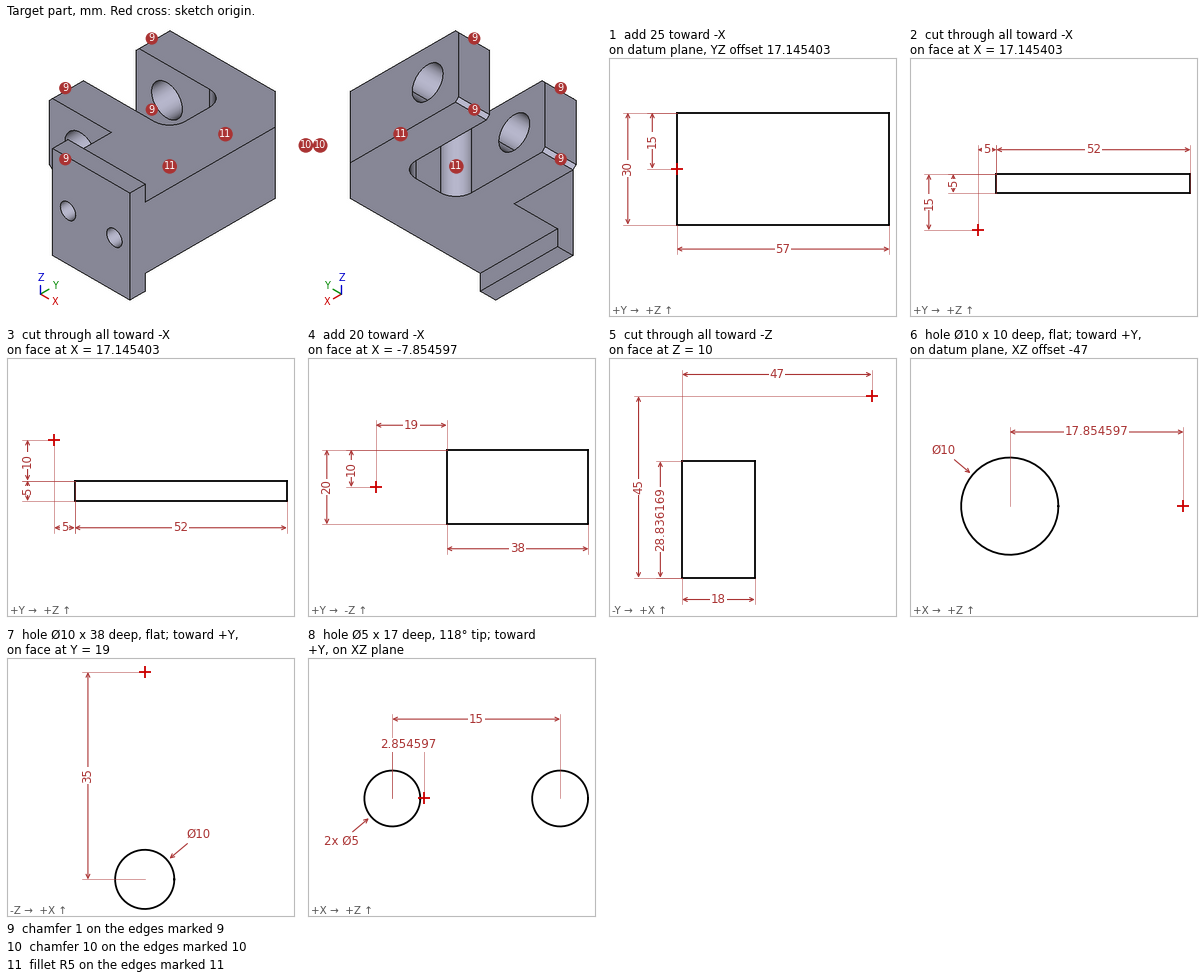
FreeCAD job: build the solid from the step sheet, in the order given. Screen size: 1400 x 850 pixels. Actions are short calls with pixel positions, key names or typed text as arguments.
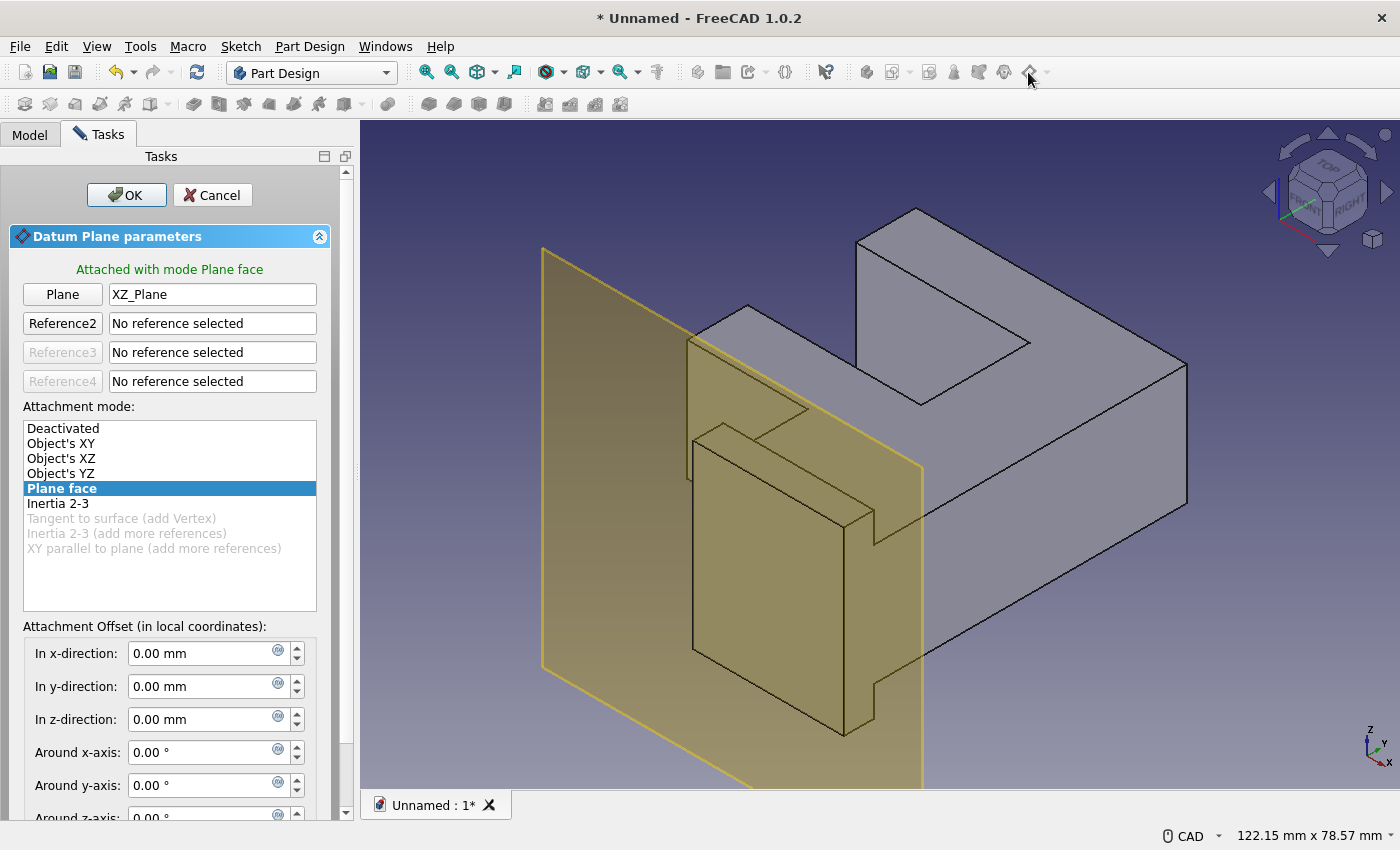
triple_click(210, 720)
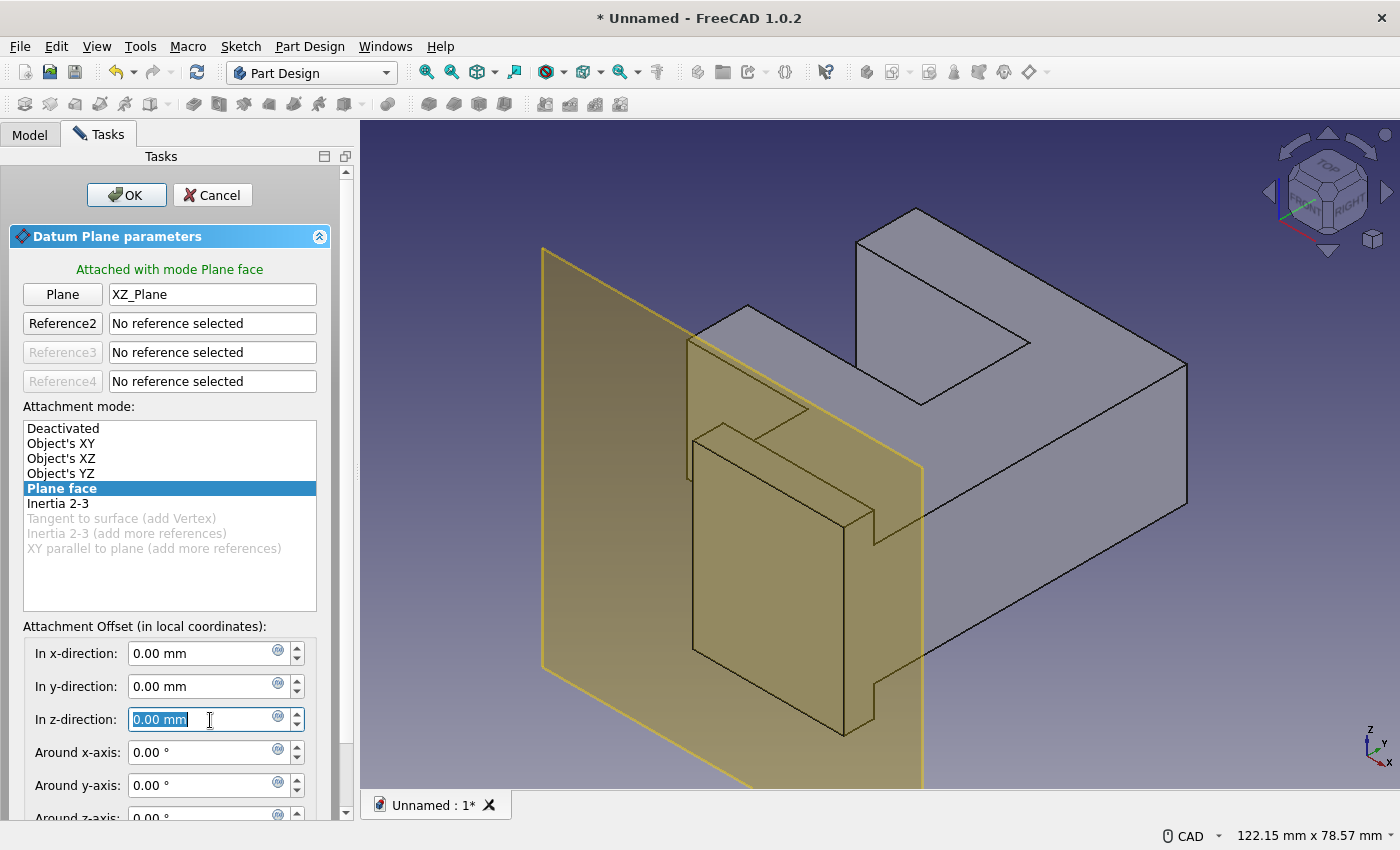
text(-47)
key(Tab)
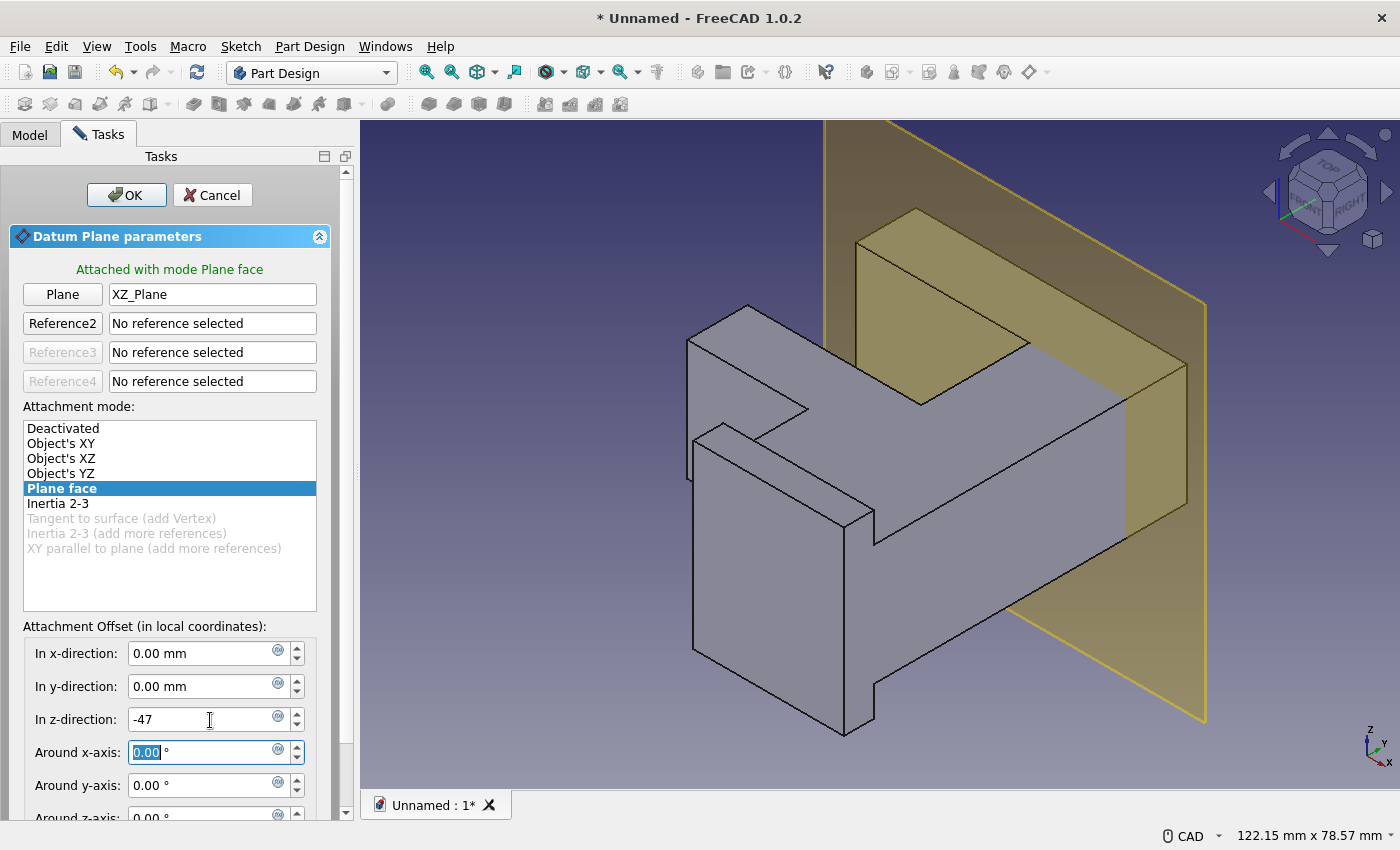
click(127, 195)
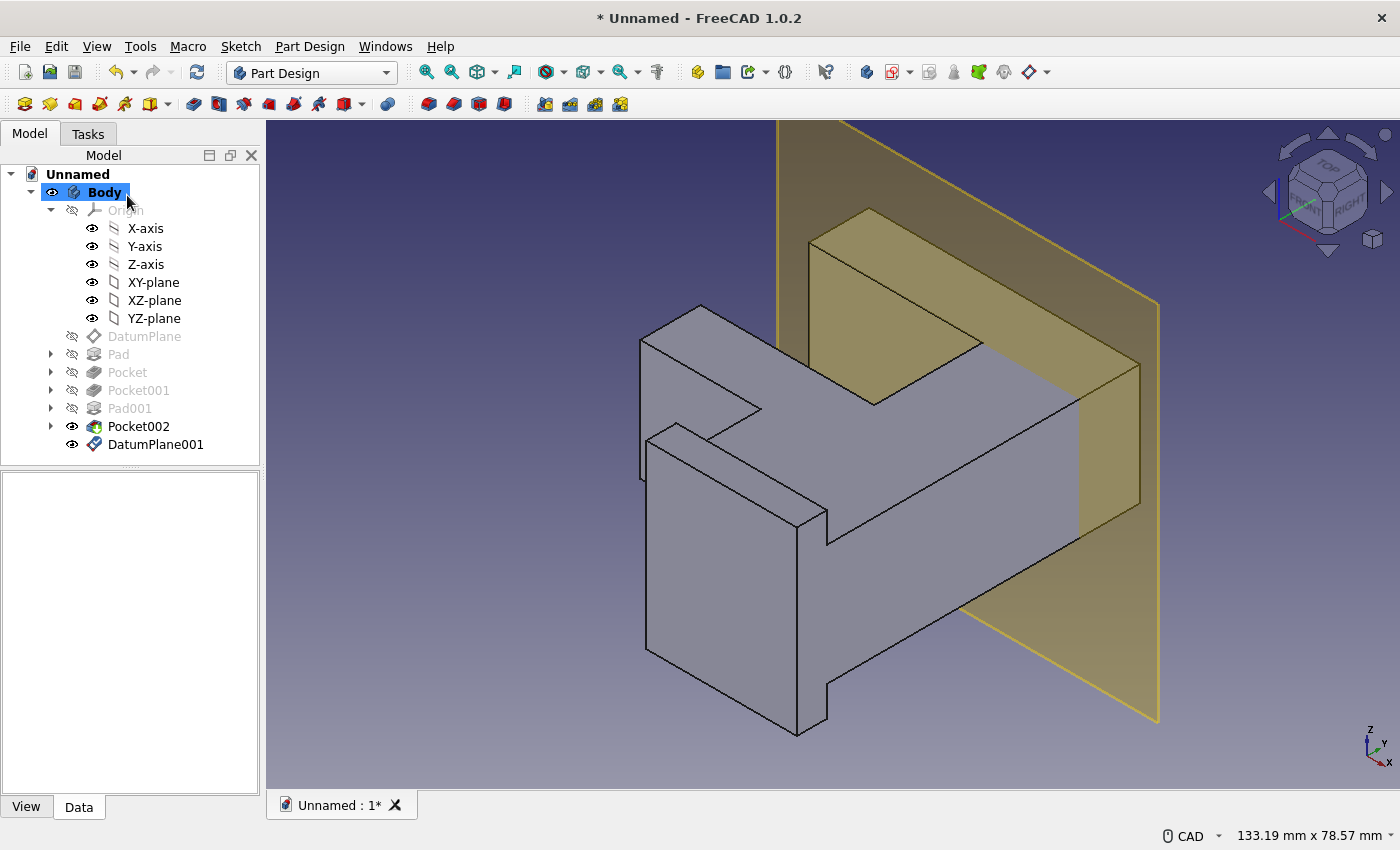
click(117, 444)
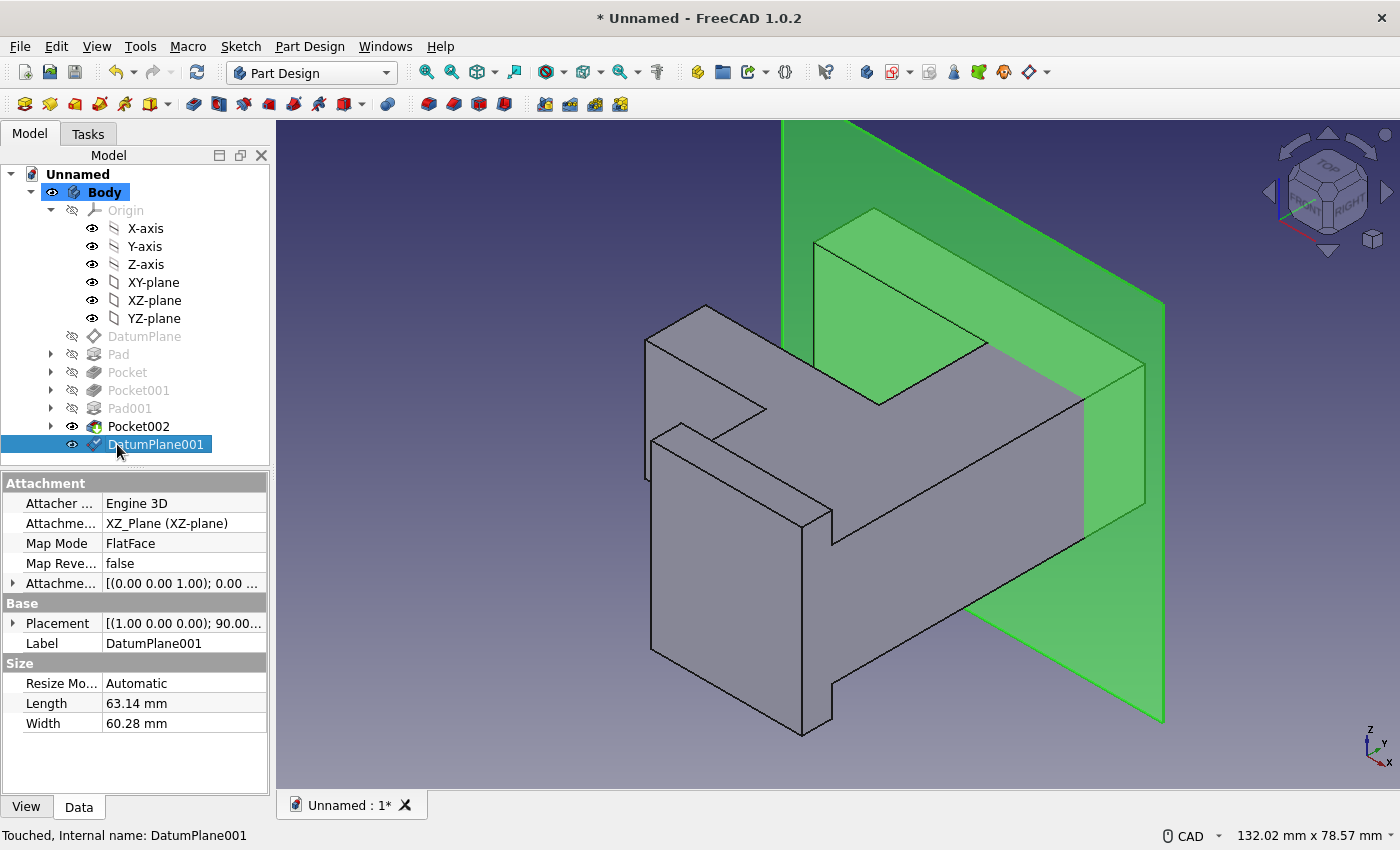
click(892, 72)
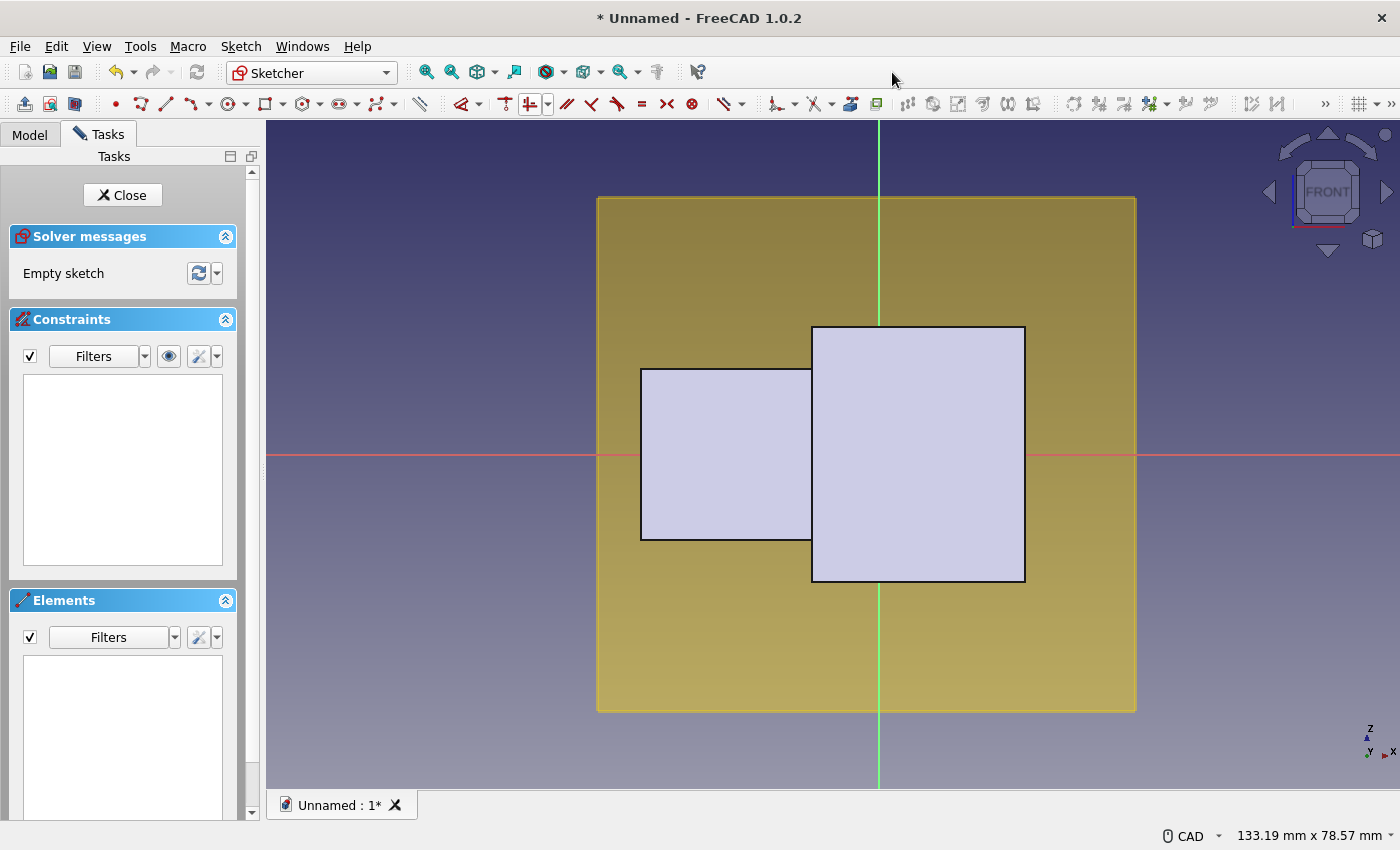
click(75, 104)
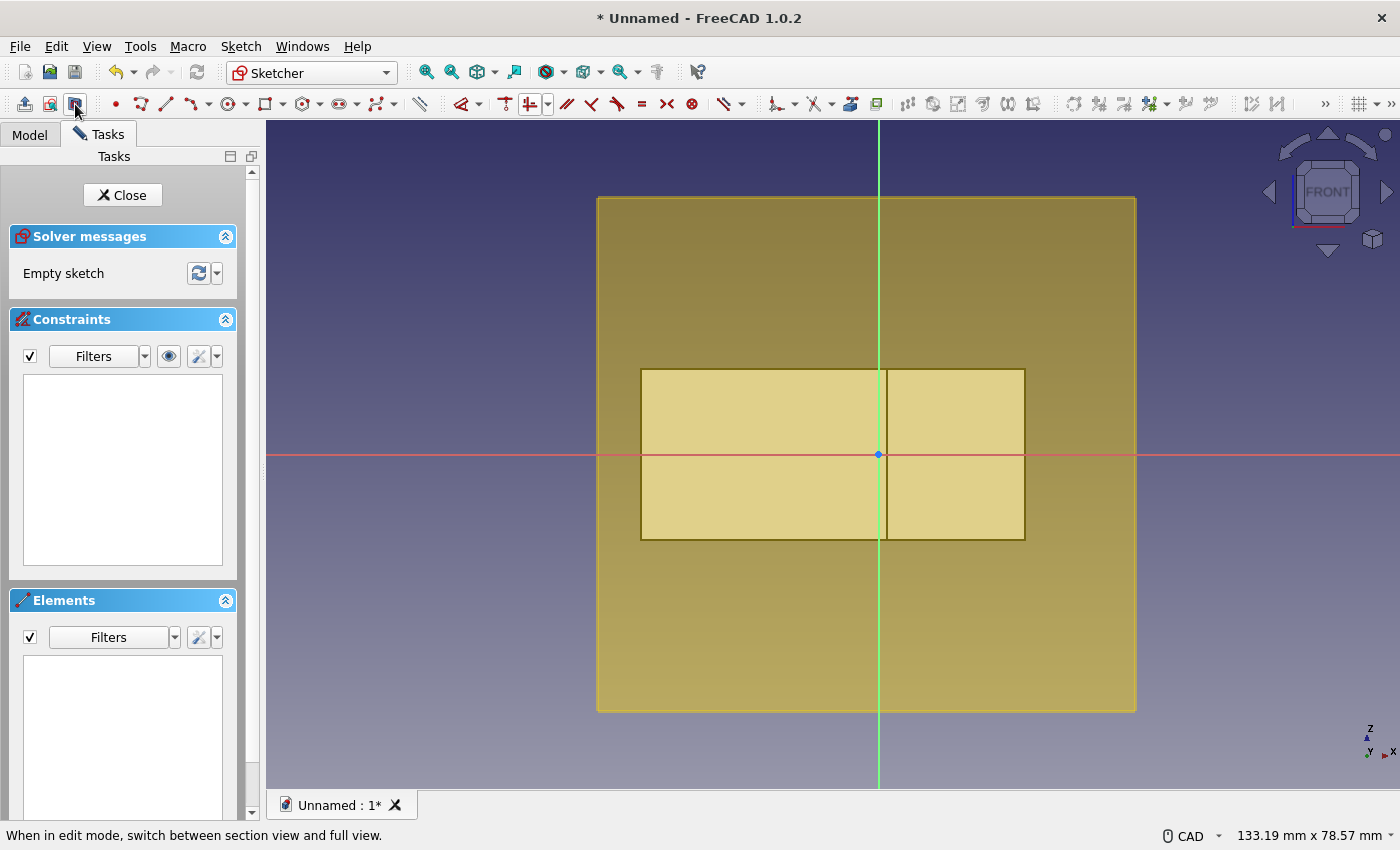
scroll(789, 455, up, 6)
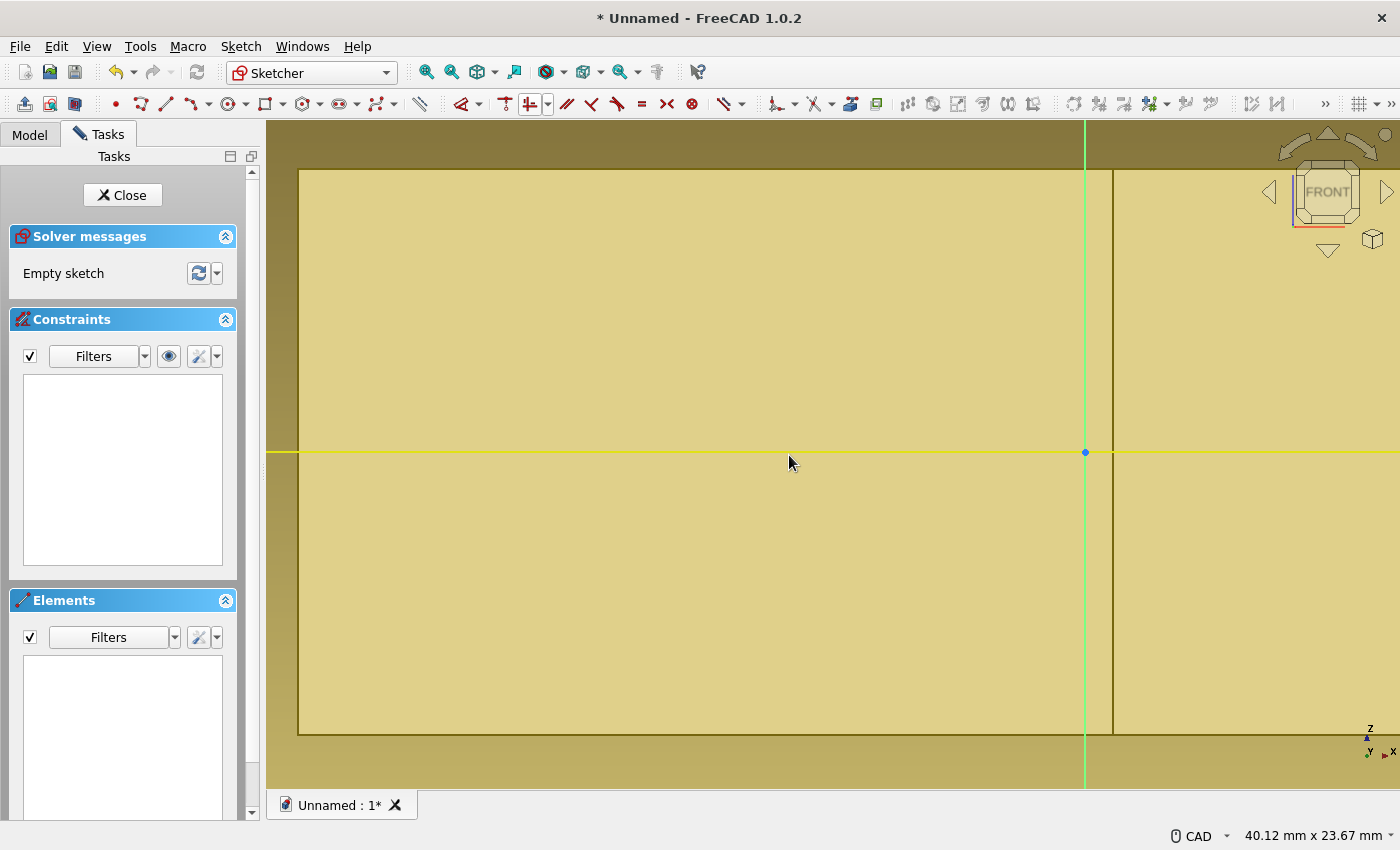
click(228, 104)